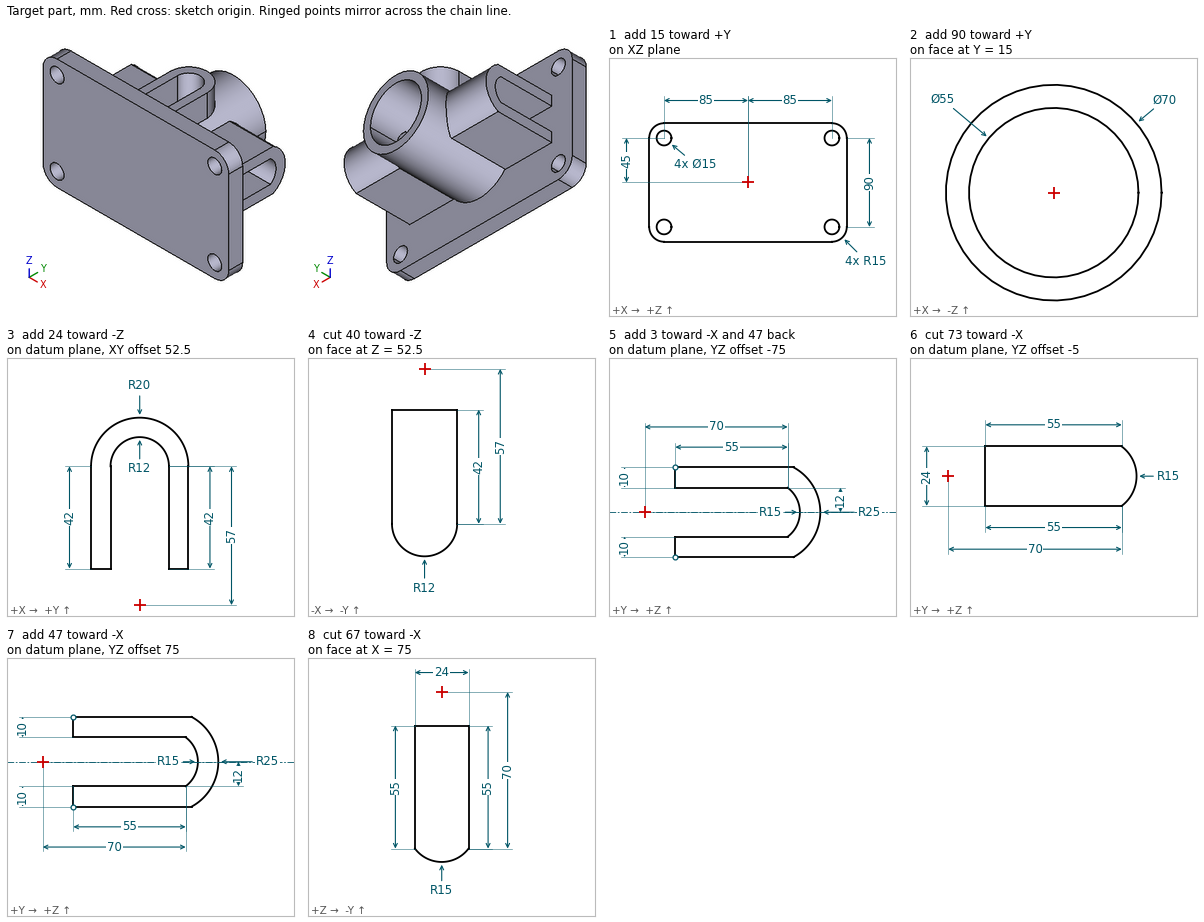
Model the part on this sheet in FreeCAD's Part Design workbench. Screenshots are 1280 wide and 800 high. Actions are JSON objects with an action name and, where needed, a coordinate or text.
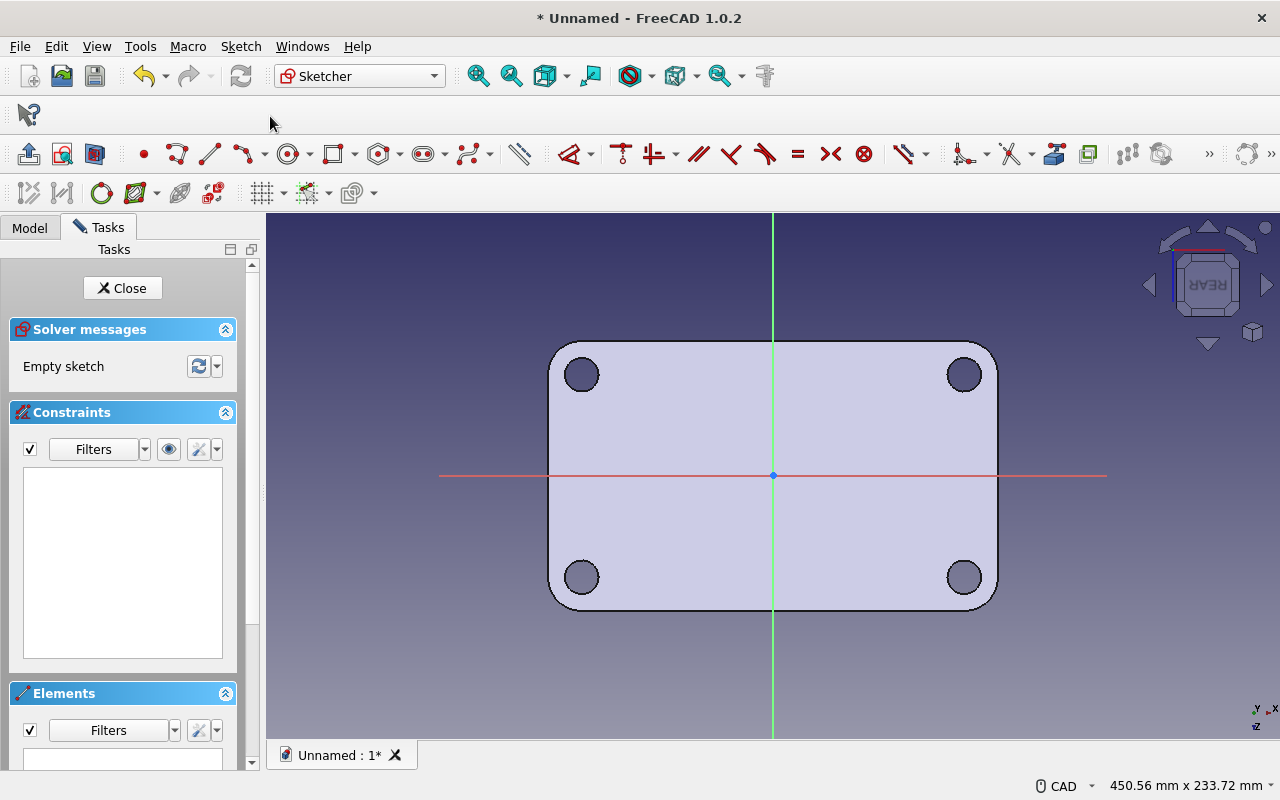
{"action": "scroll", "coordinate": [829, 476], "scroll_direction": "up", "scroll_amount": 4}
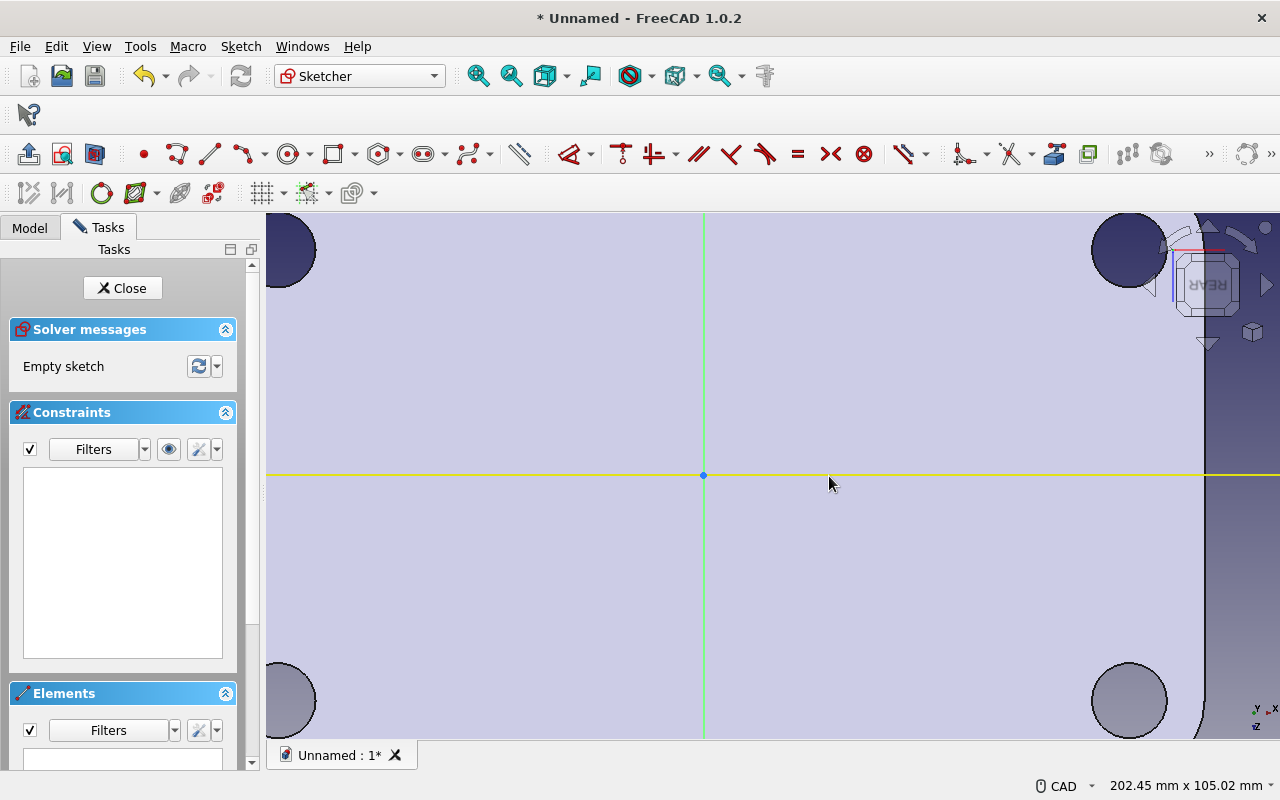
{"action": "key", "text": "g c"}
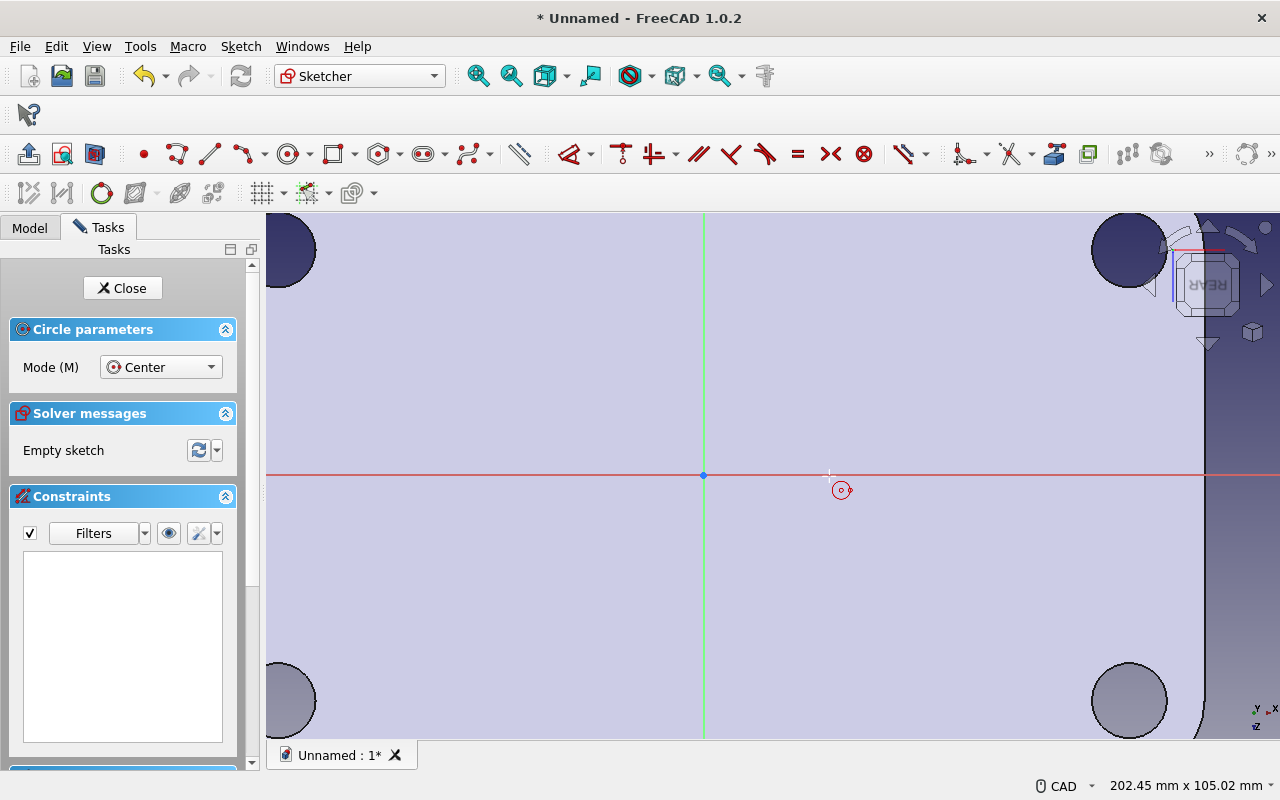
{"action": "left_click", "coordinate": [704, 475]}
{"action": "mouse_move", "coordinate": [828, 351]}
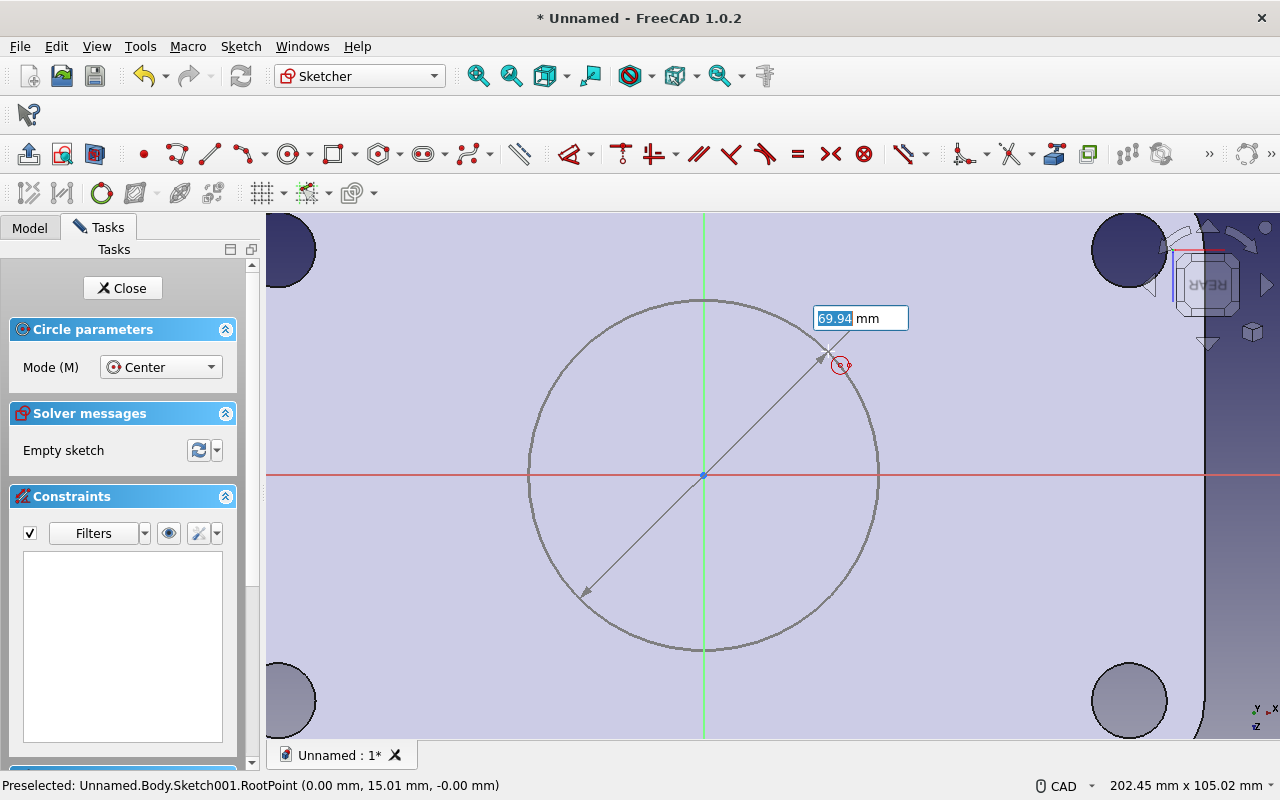
{"action": "type", "text": "70"}
{"action": "key", "text": "Return"}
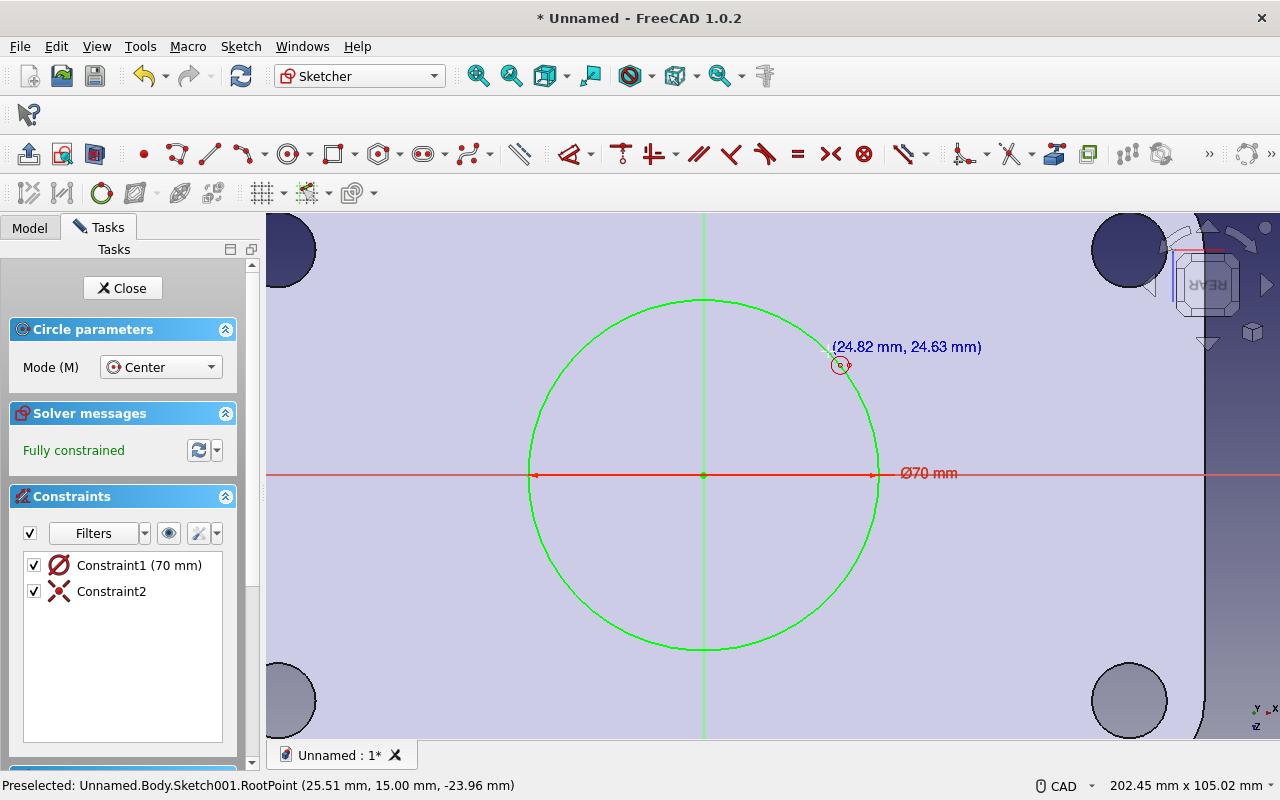
{"action": "left_click", "coordinate": [704, 475]}
{"action": "mouse_move", "coordinate": [801, 378]}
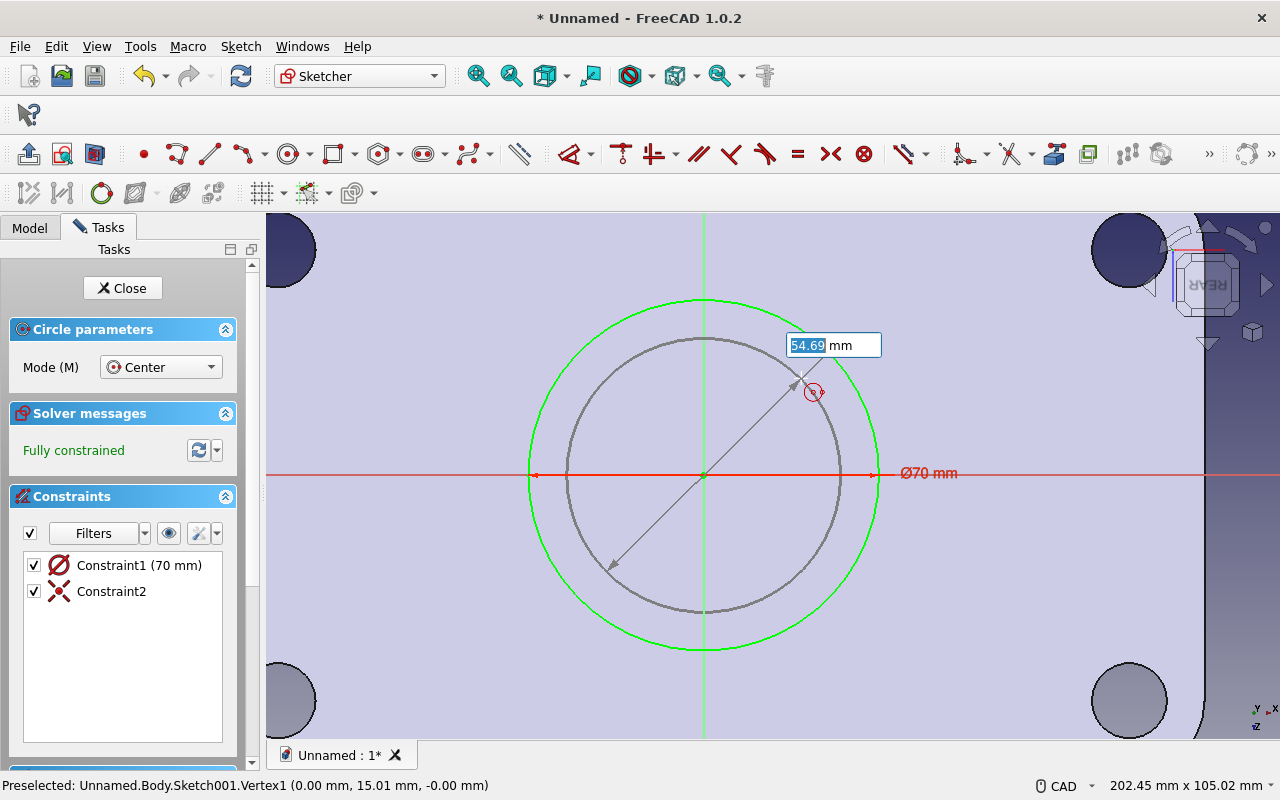
{"action": "type", "text": "55"}
{"action": "key", "text": "Return"}
{"action": "key", "text": "Escape"}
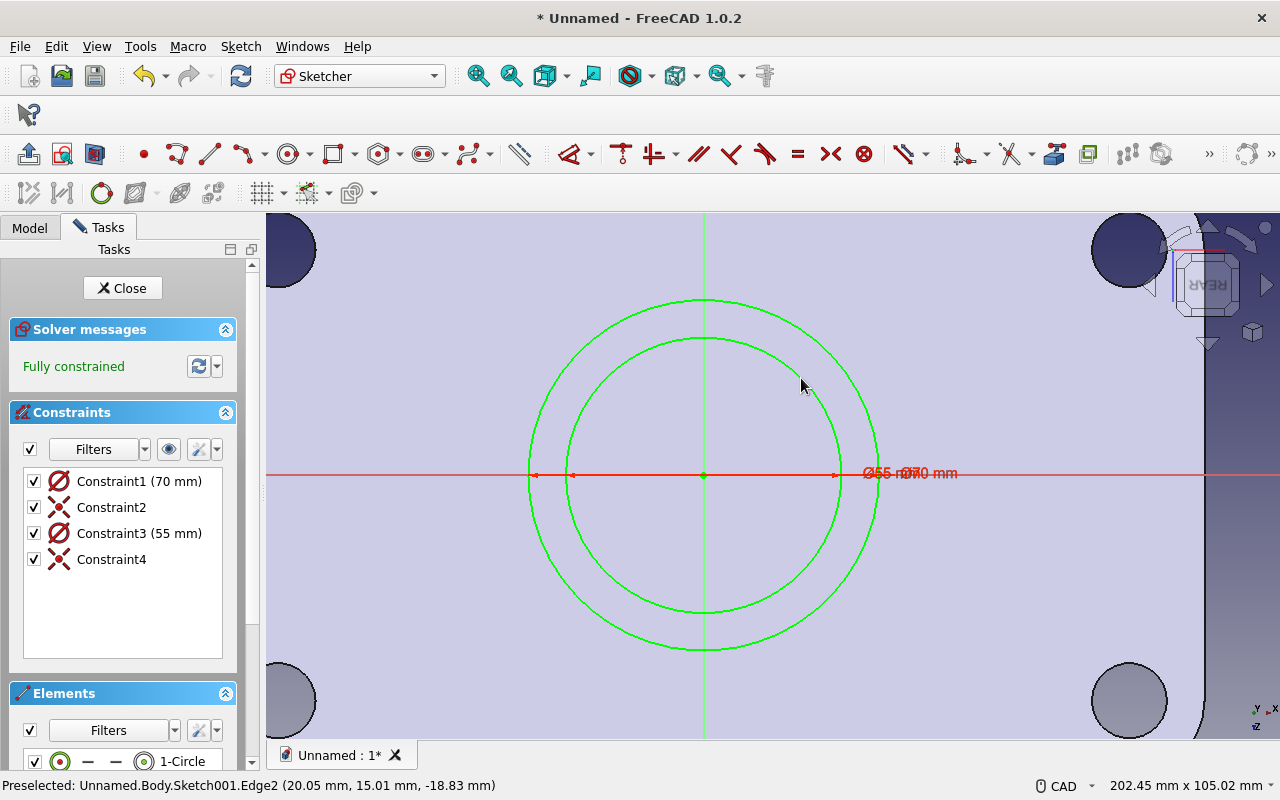
{"action": "left_click", "coordinate": [123, 288]}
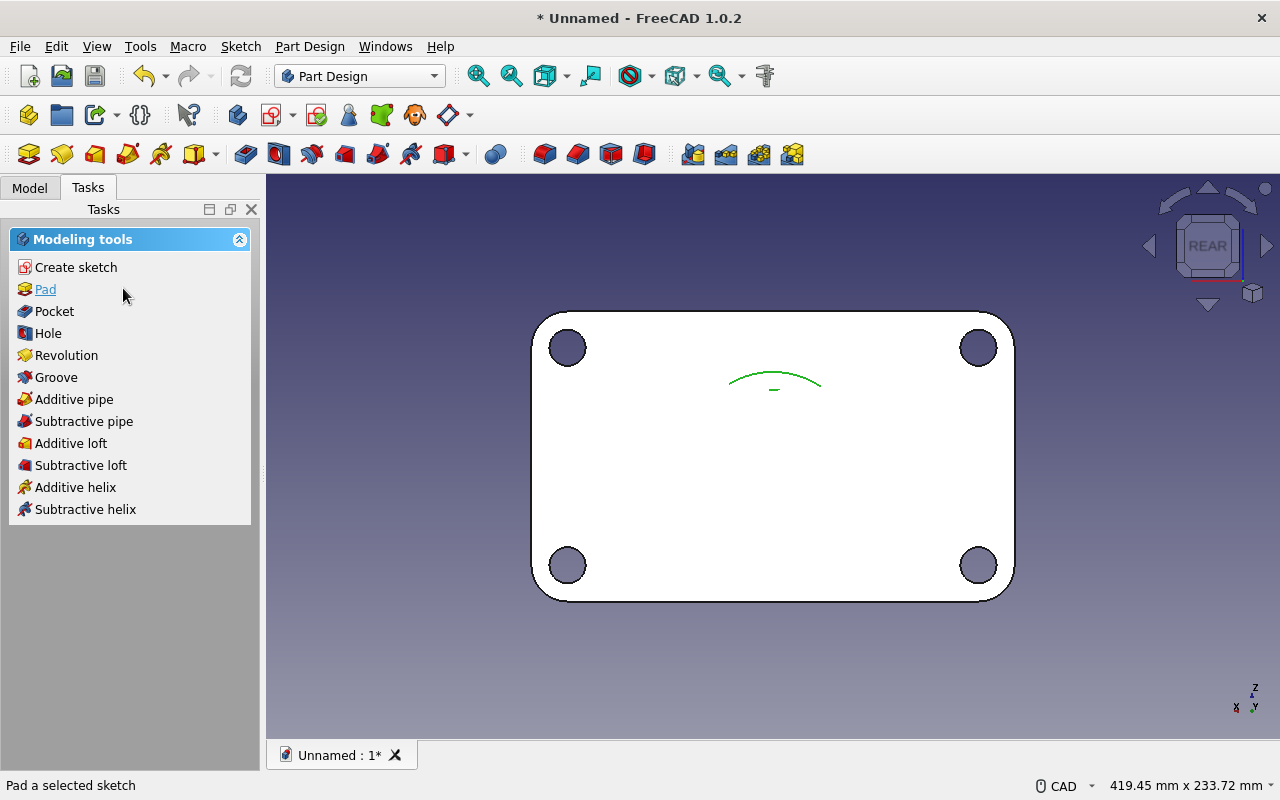
{"action": "left_click", "coordinate": [29, 154]}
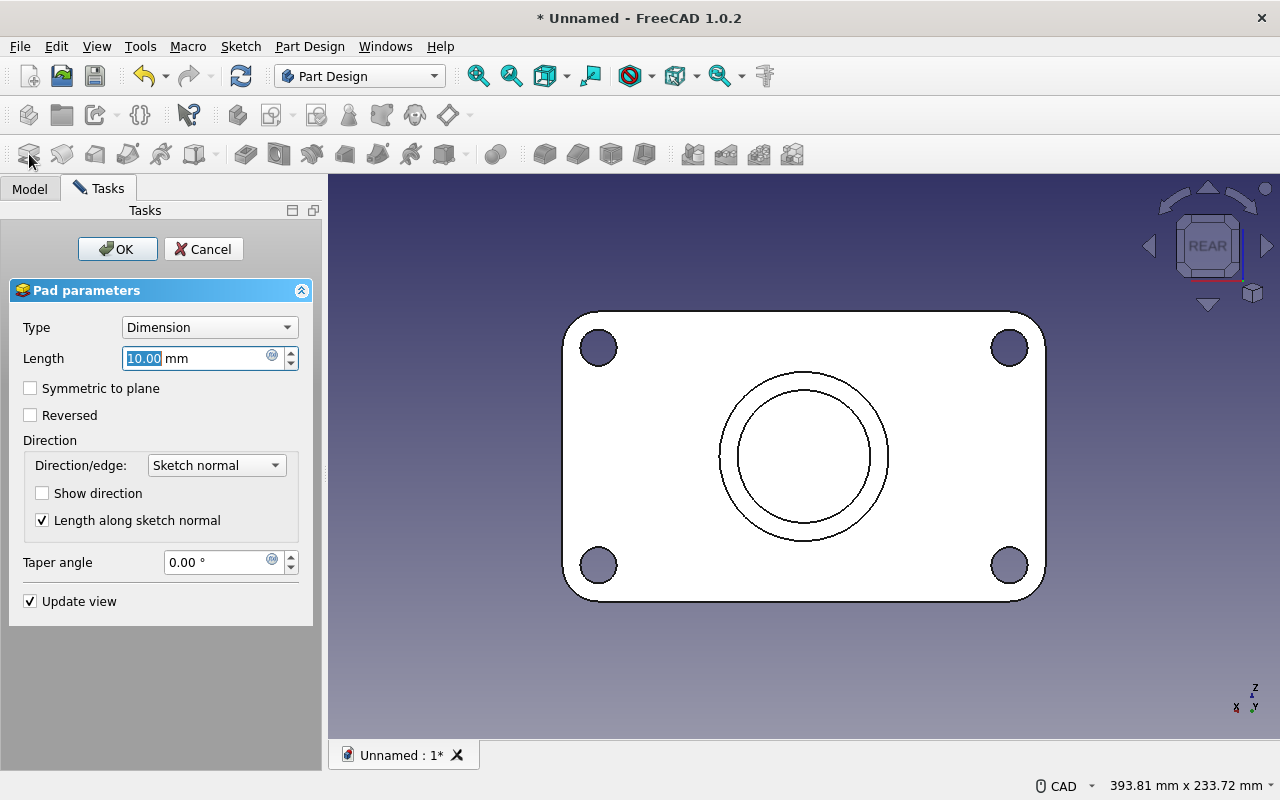
{"action": "type", "text": "90"}
{"action": "key", "text": "Tab"}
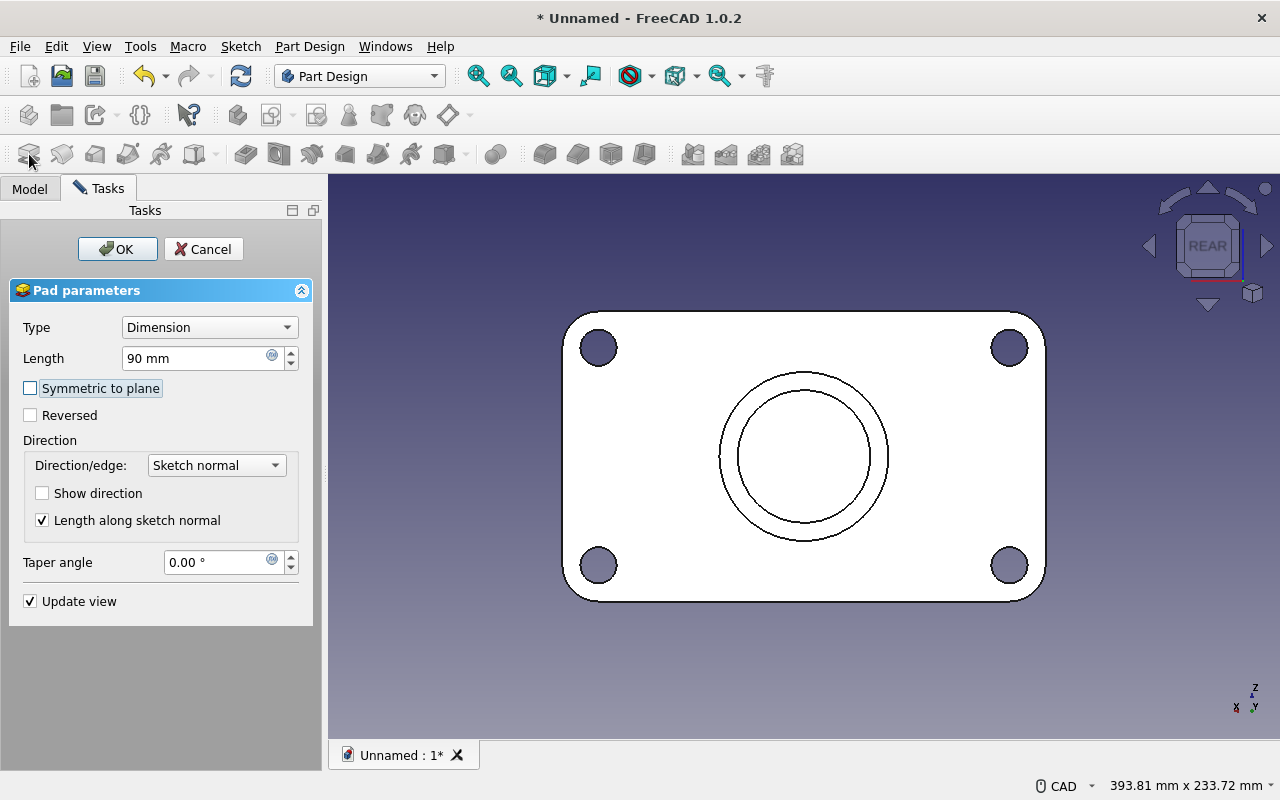
{"action": "left_click", "coordinate": [118, 249]}